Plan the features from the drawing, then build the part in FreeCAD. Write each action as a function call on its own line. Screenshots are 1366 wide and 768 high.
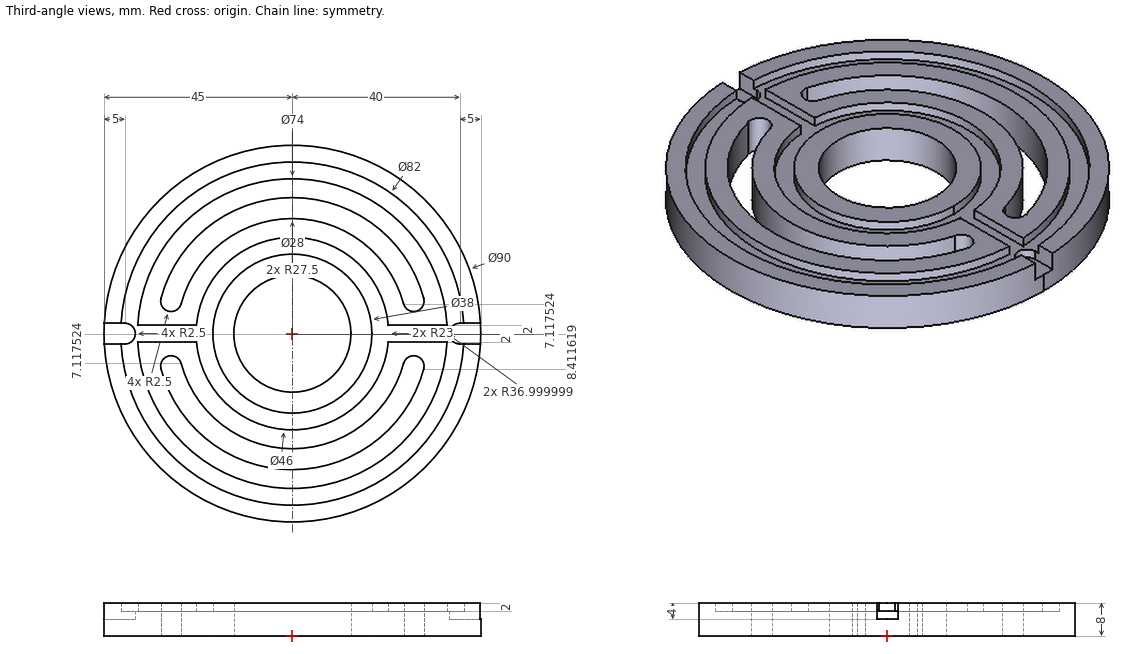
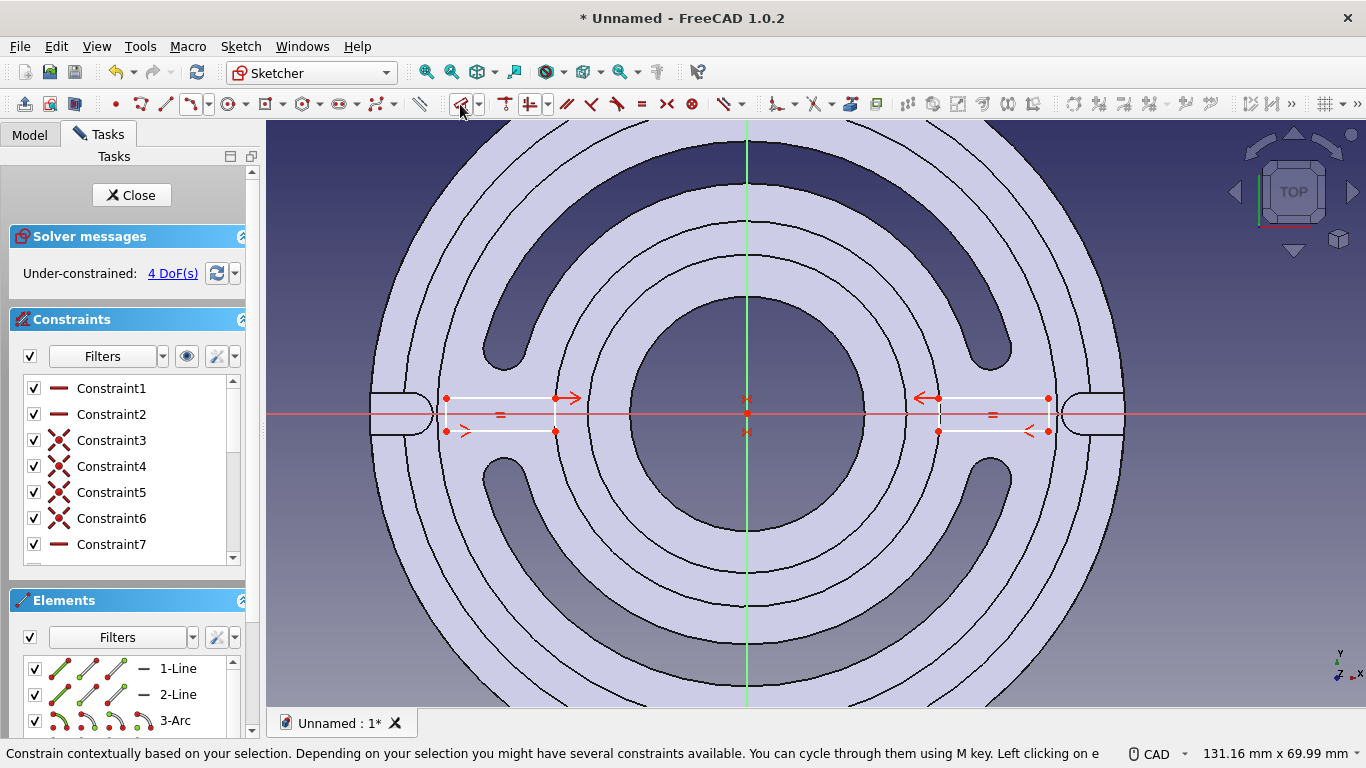
click(1049, 415)
click(1040, 575)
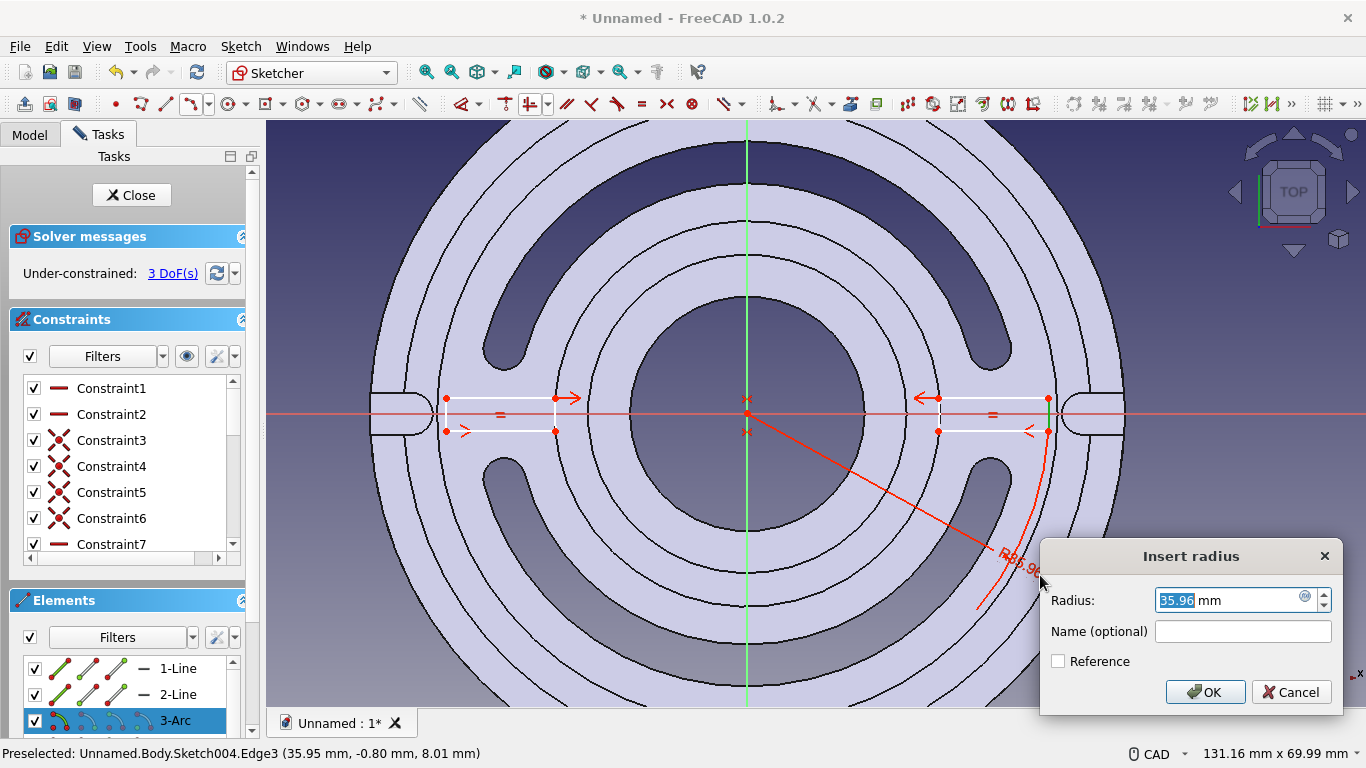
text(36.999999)
key(Return)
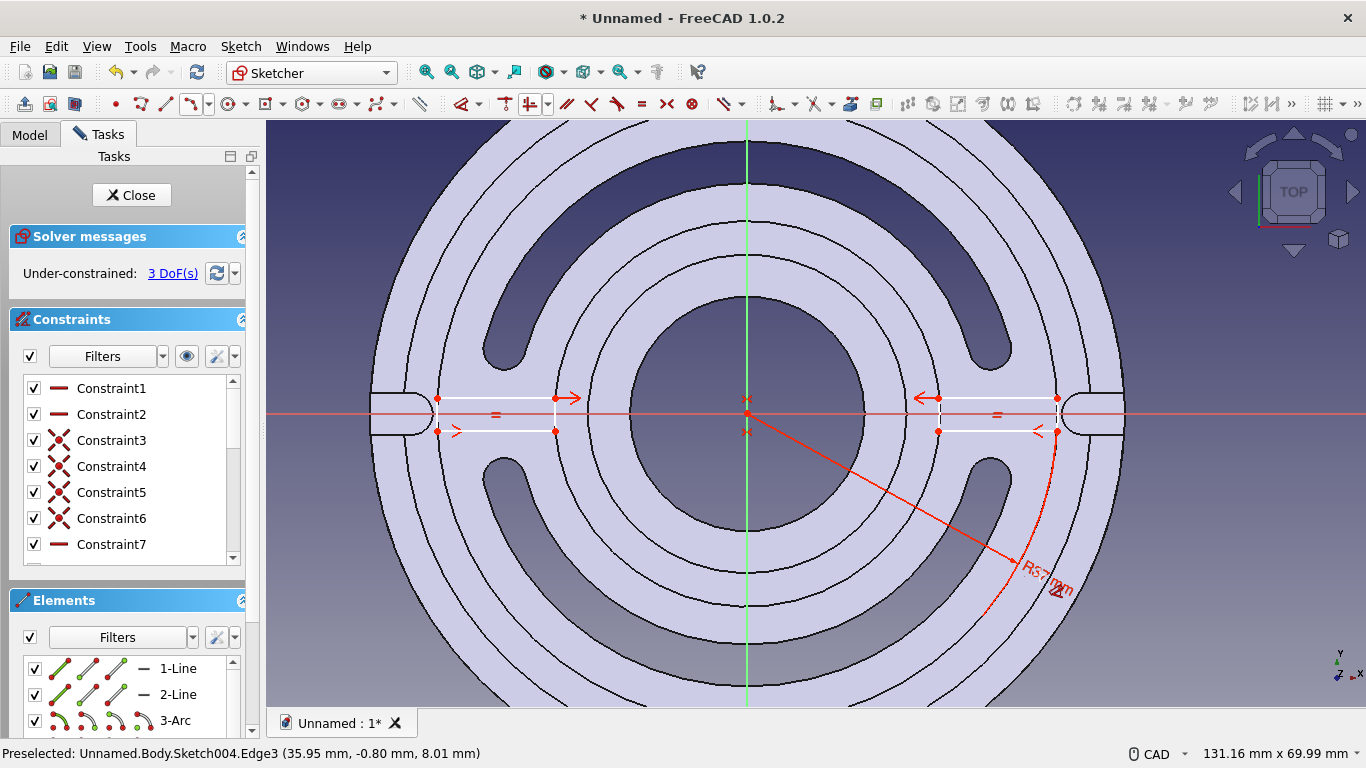
click(940, 415)
click(944, 523)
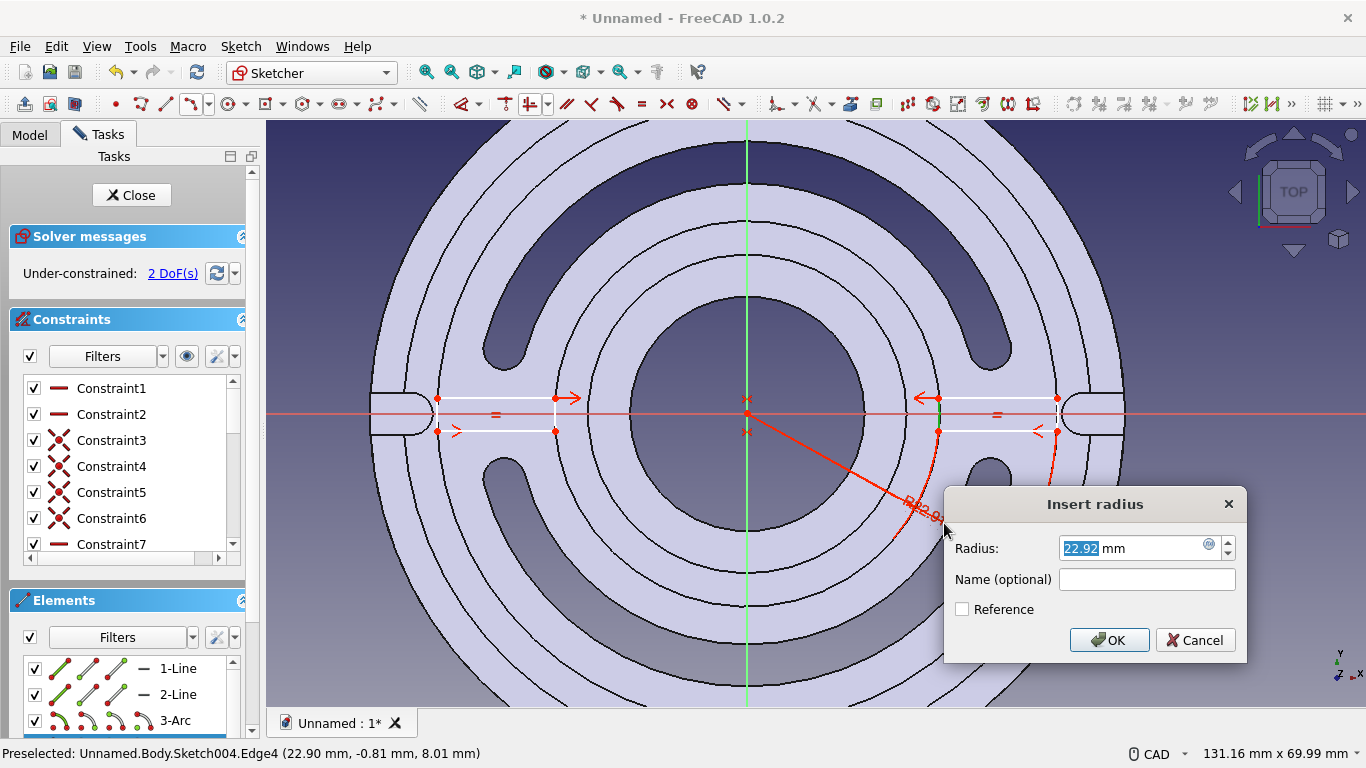
text(23)
key(Return)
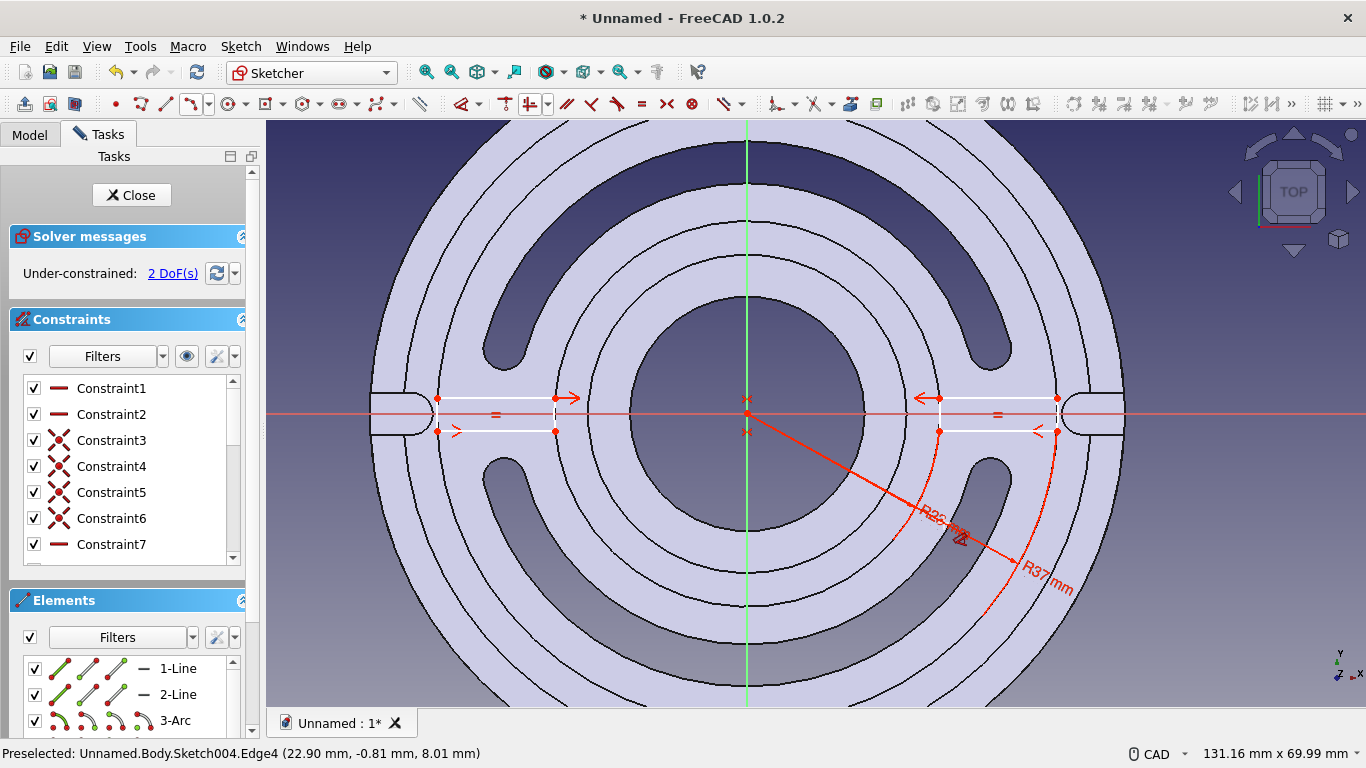
scroll(939, 431, up, 5)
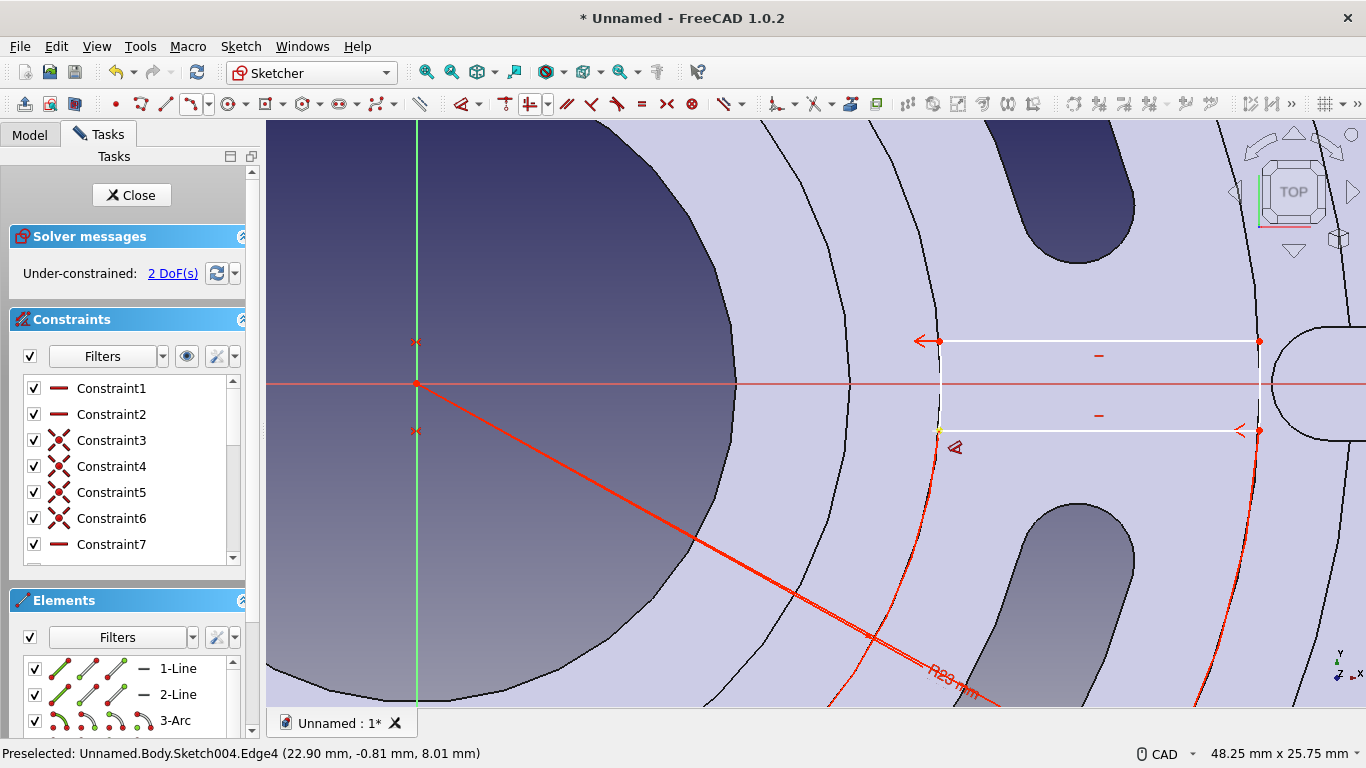
click(939, 431)
click(973, 407)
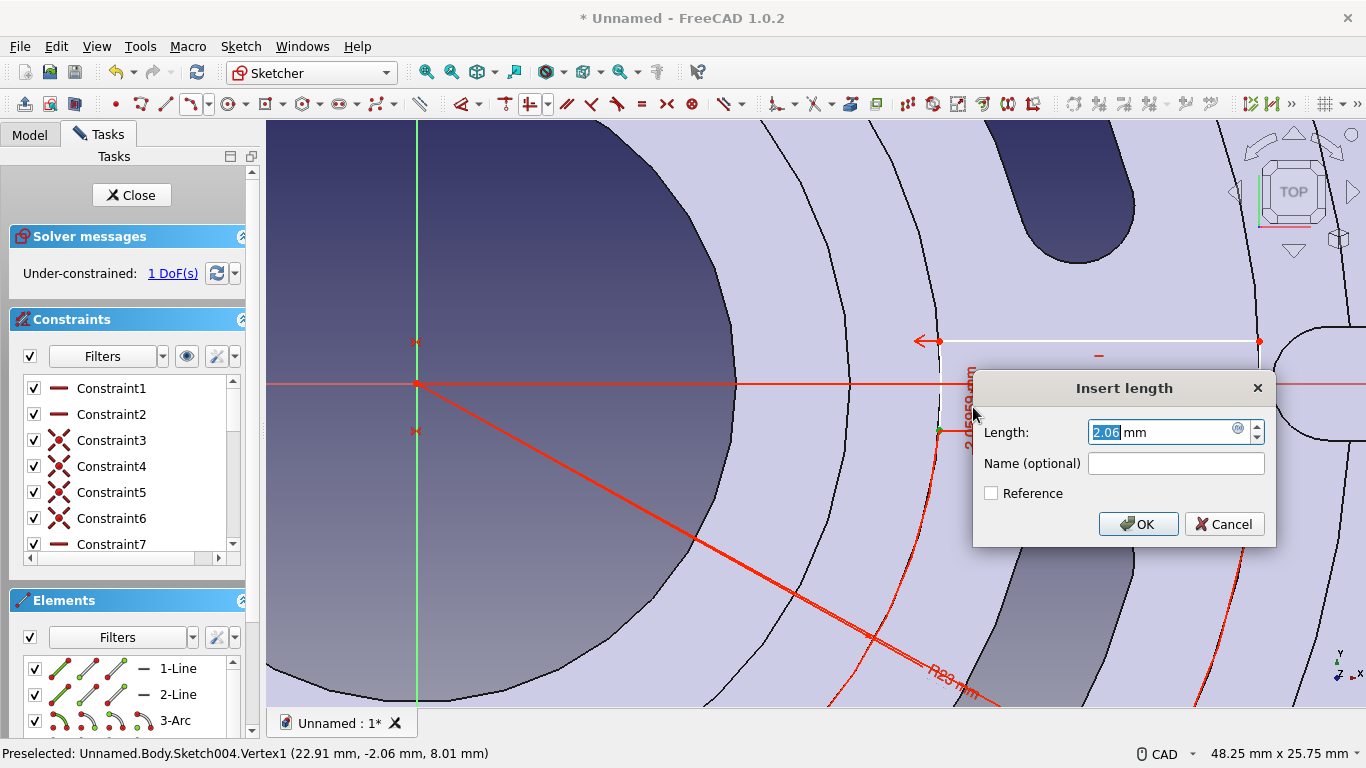
text(2)
key(Return)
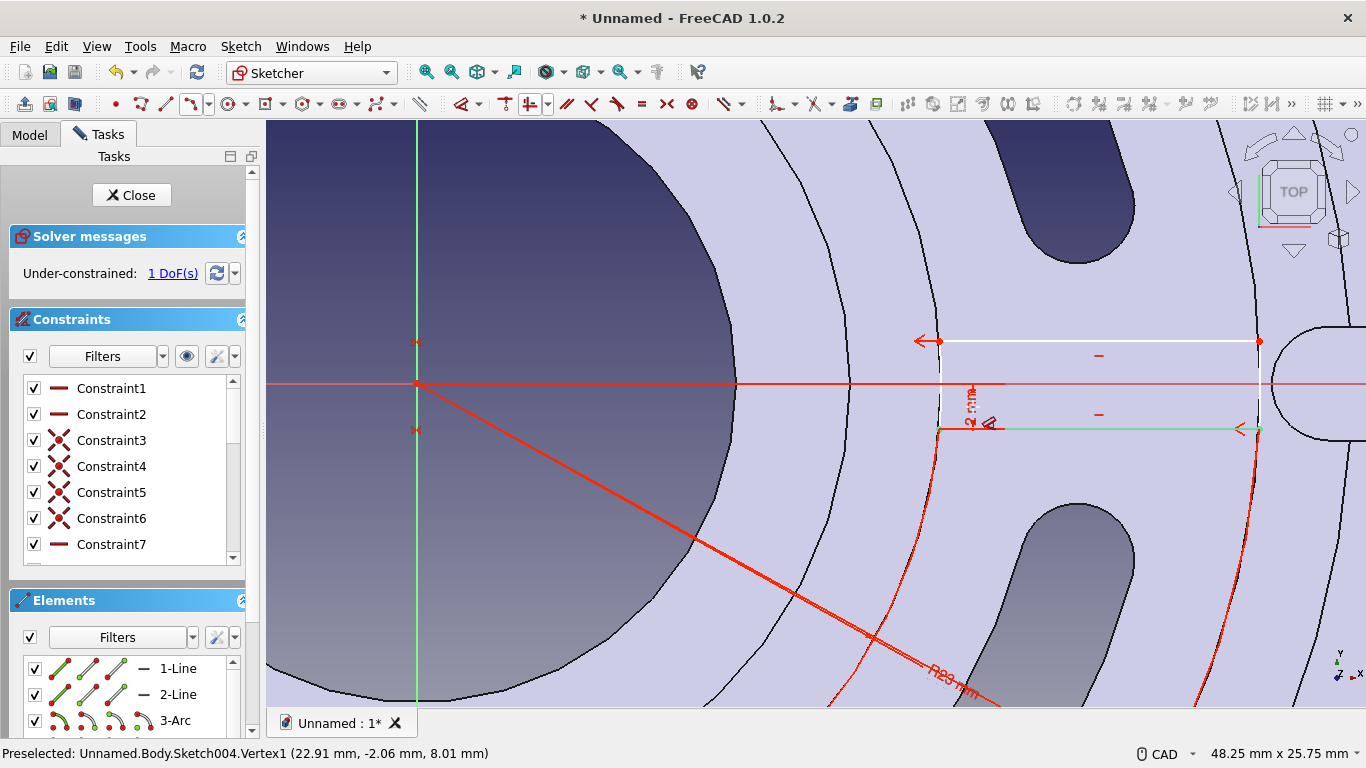
scroll(940, 431, down, 5)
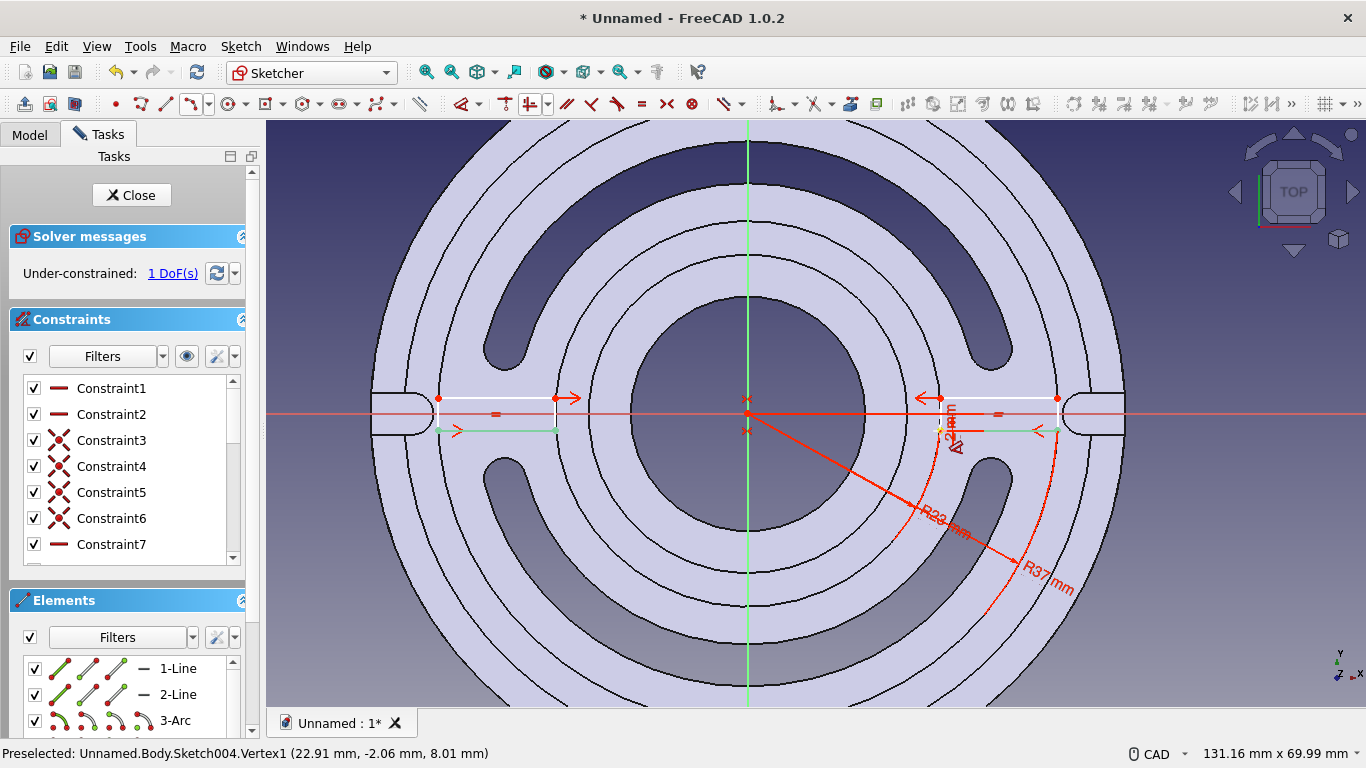
scroll(1058, 398, up, 5)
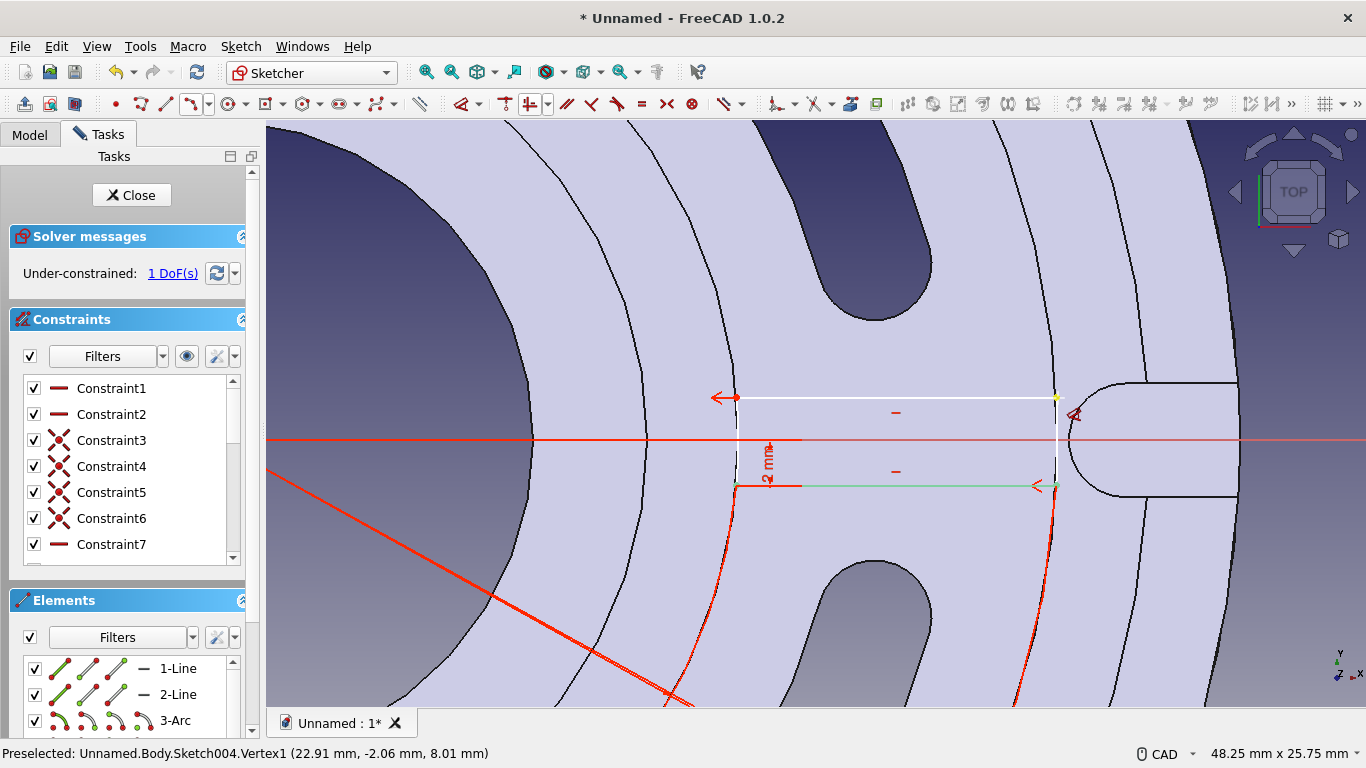
click(1056, 398)
click(1090, 419)